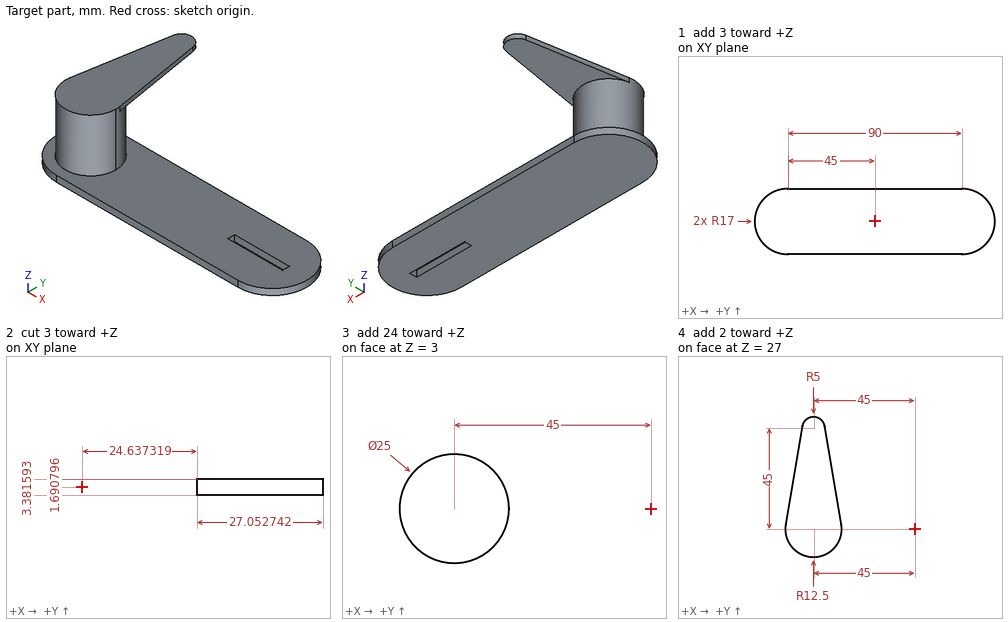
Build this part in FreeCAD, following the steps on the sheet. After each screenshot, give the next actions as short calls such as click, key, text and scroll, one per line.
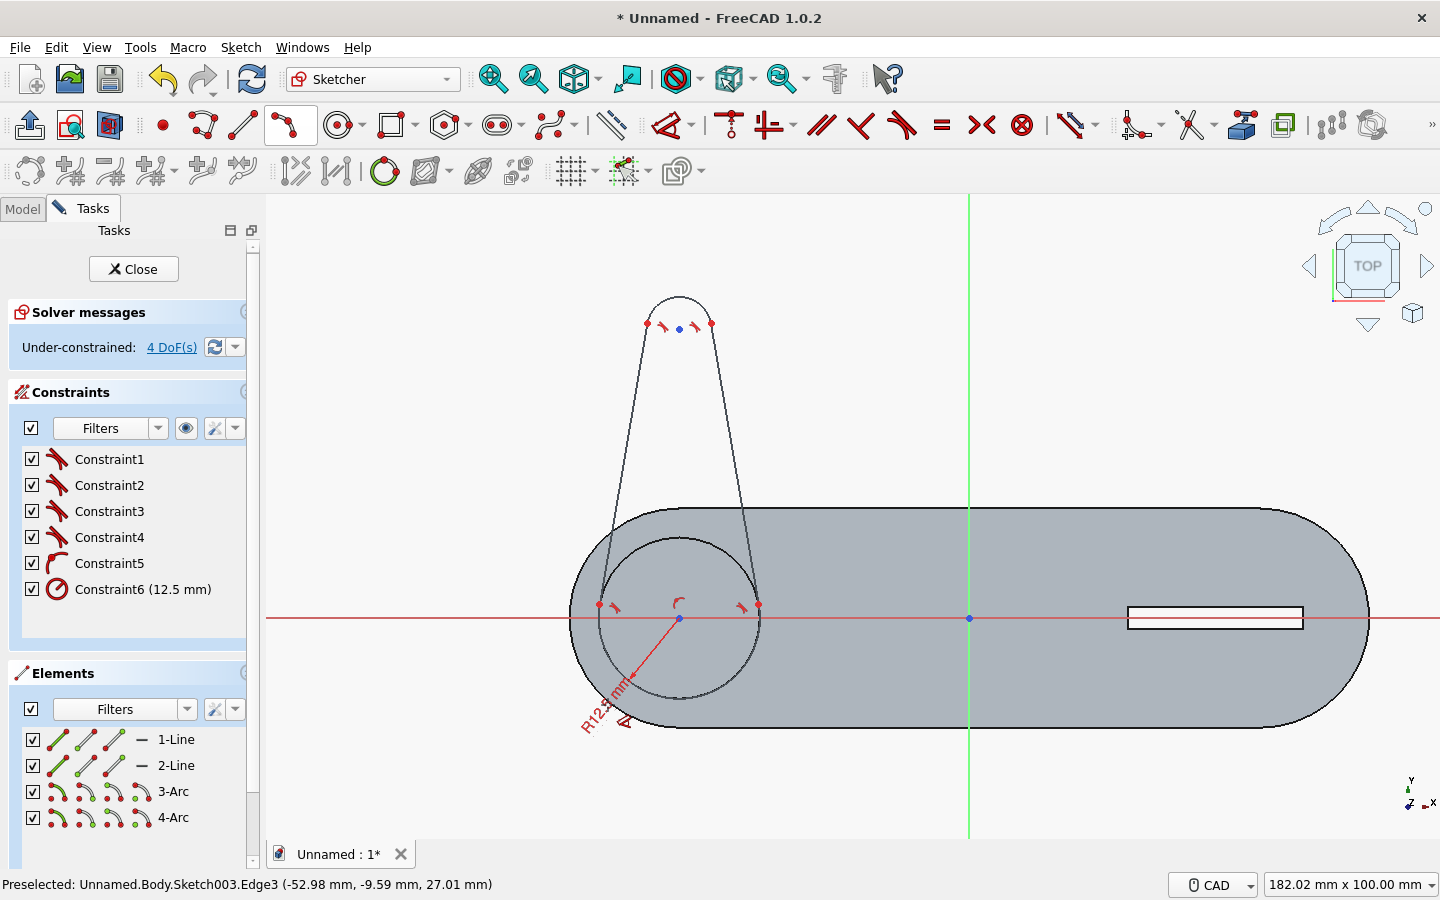
scroll(696, 302, up, 2)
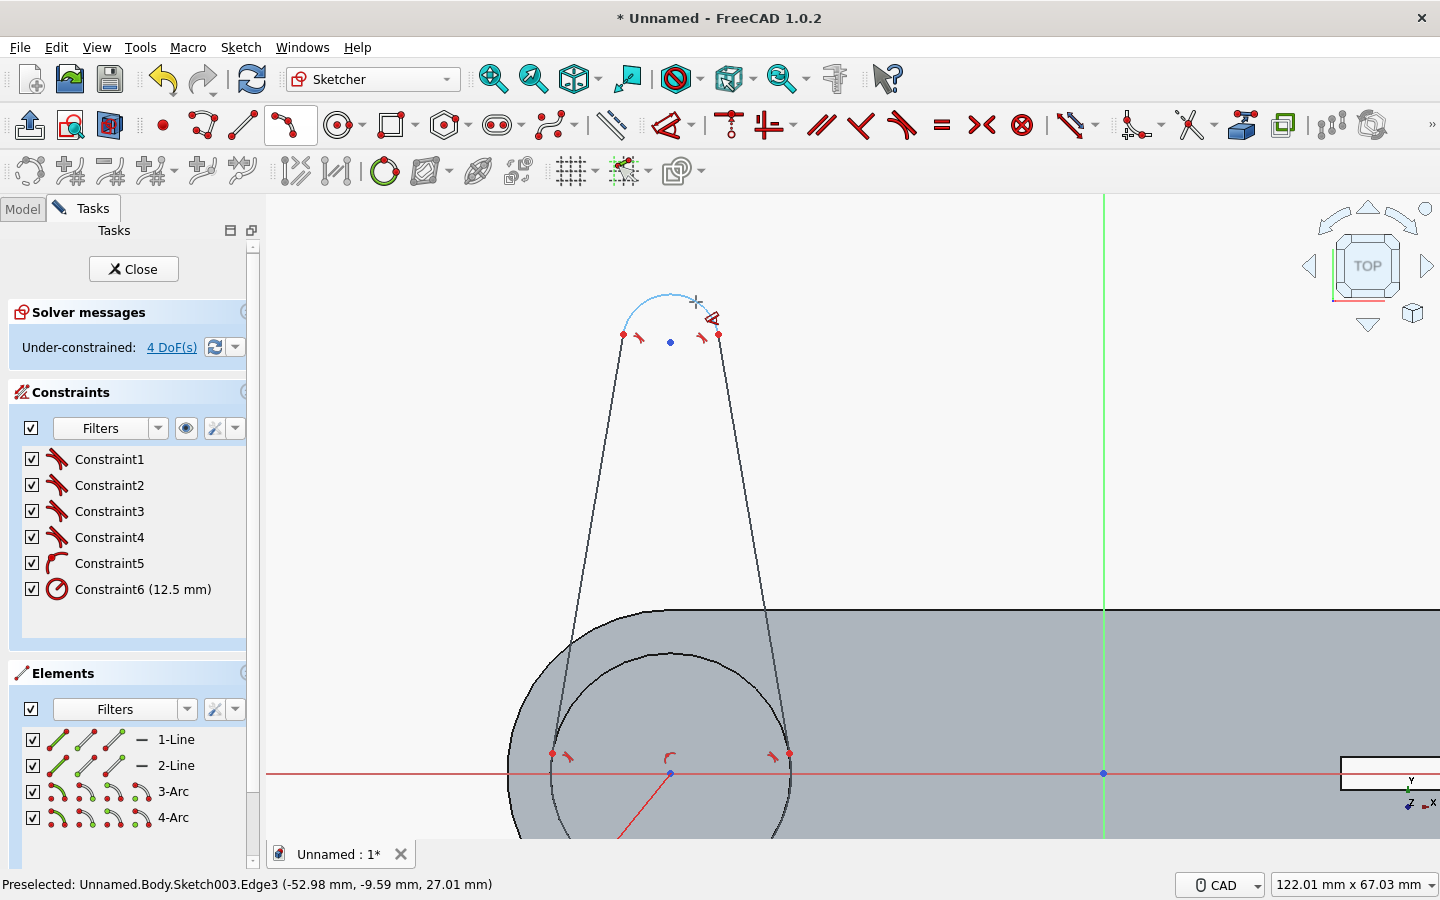
click(696, 302)
click(713, 275)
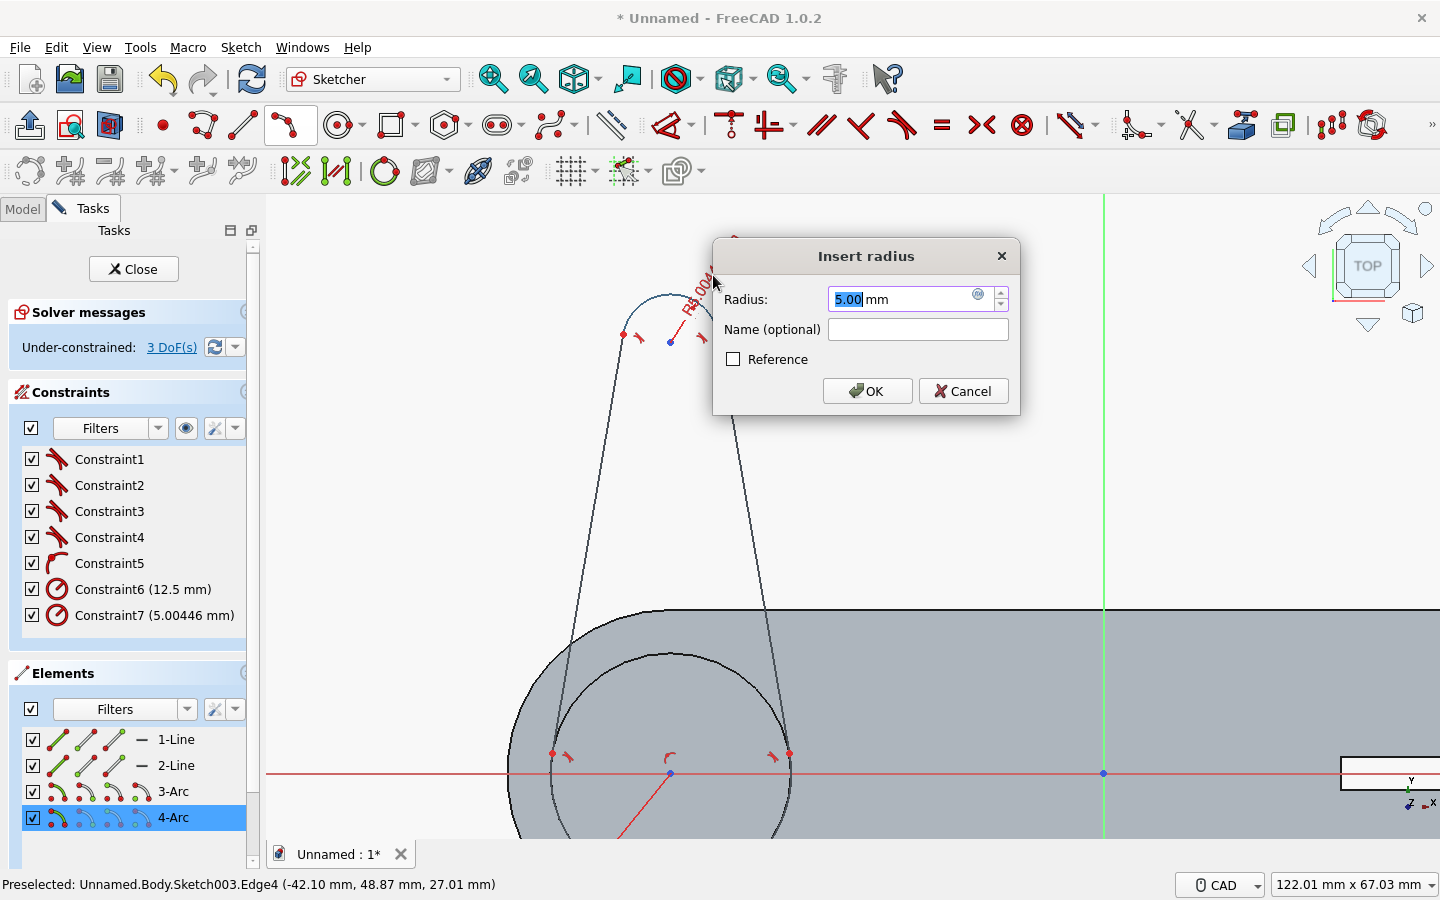
text(5)
key(Return)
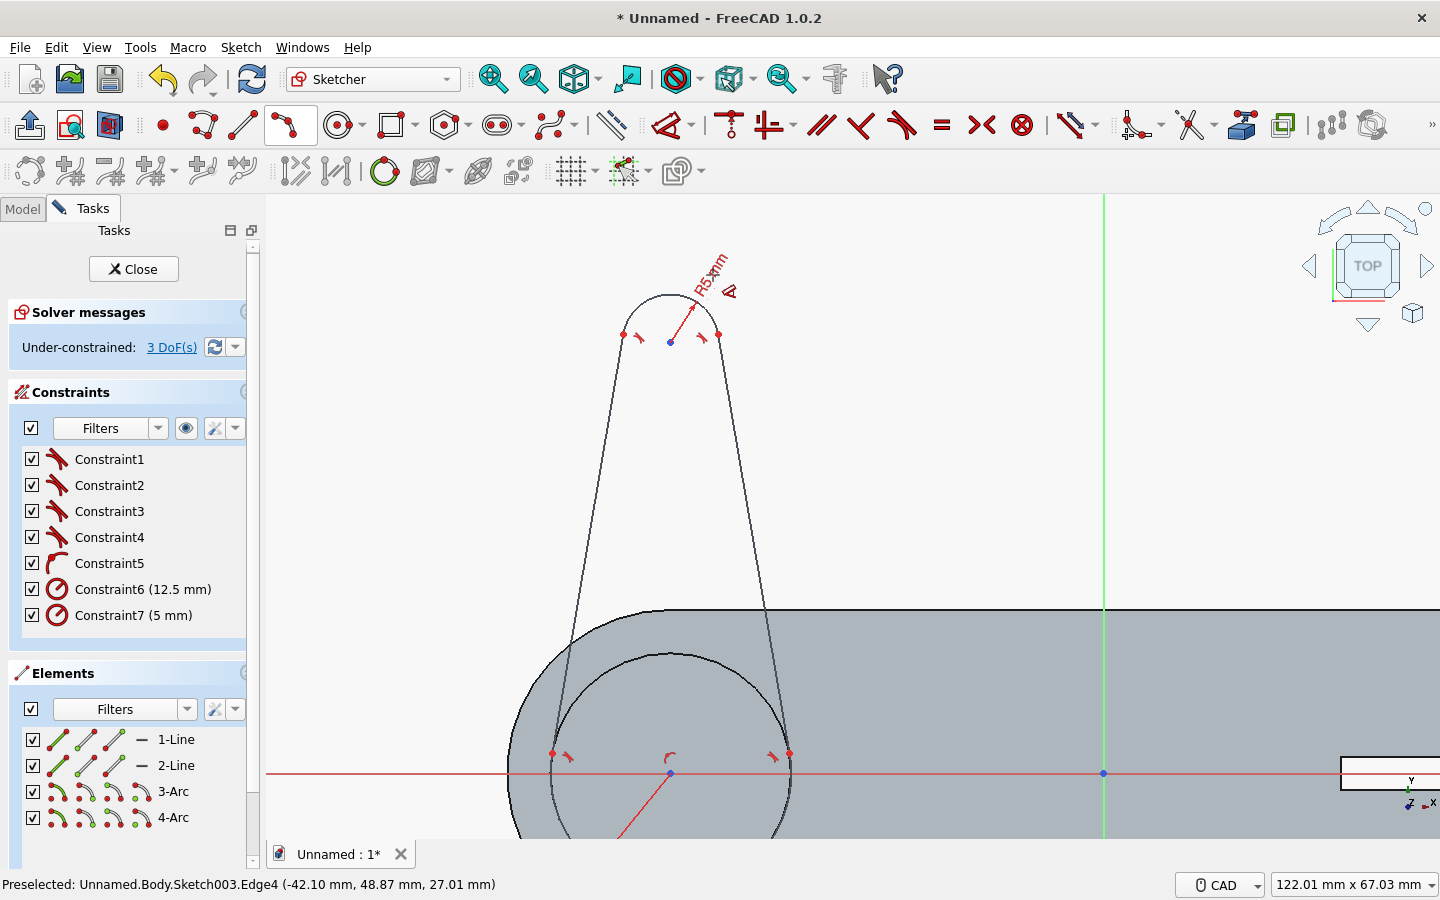
click(671, 774)
click(887, 808)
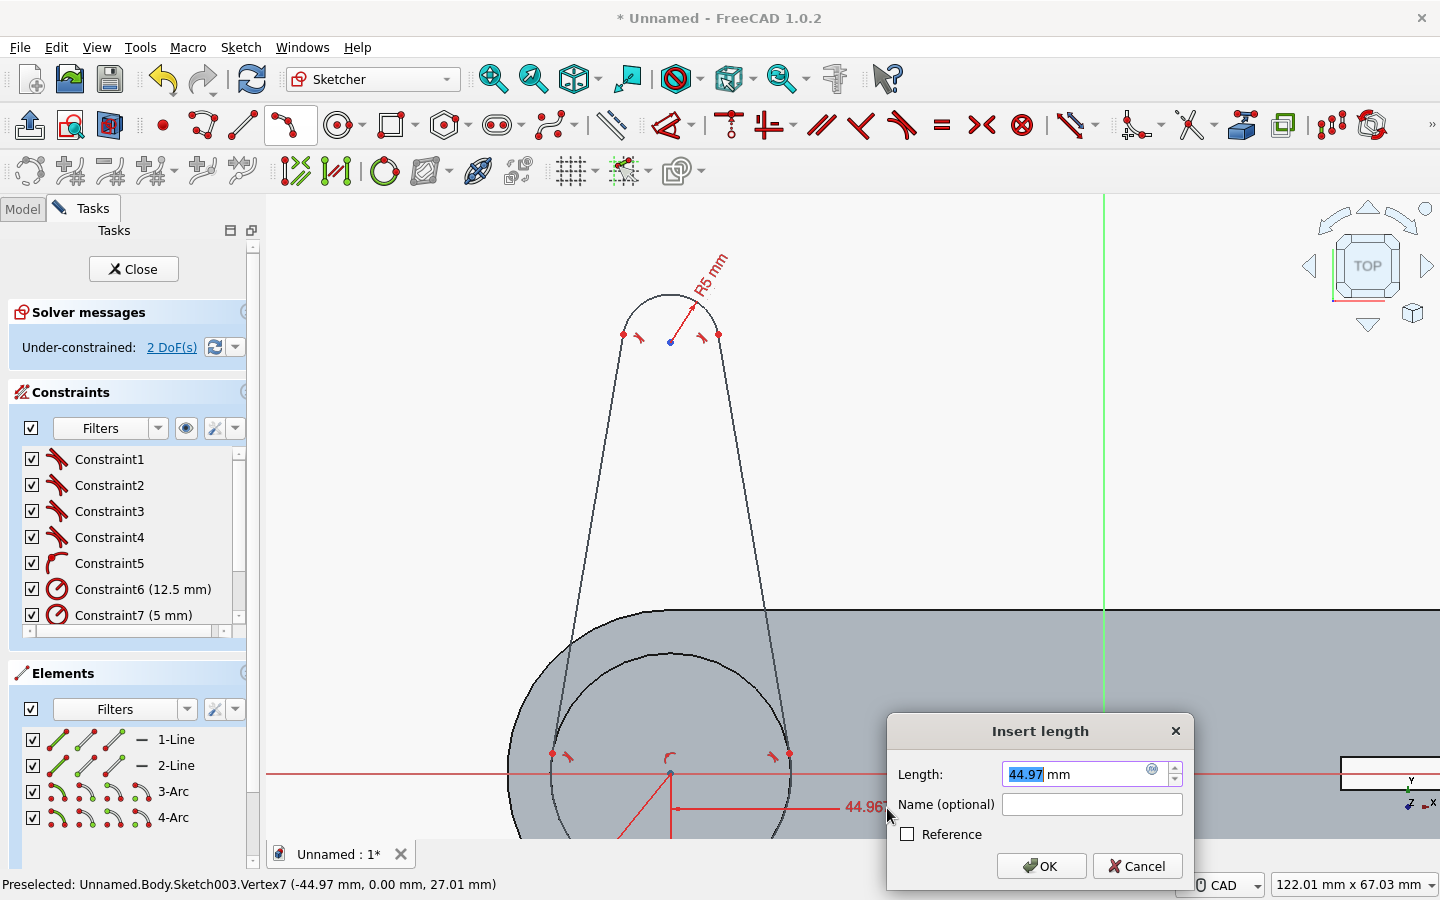
text(45)
key(Return)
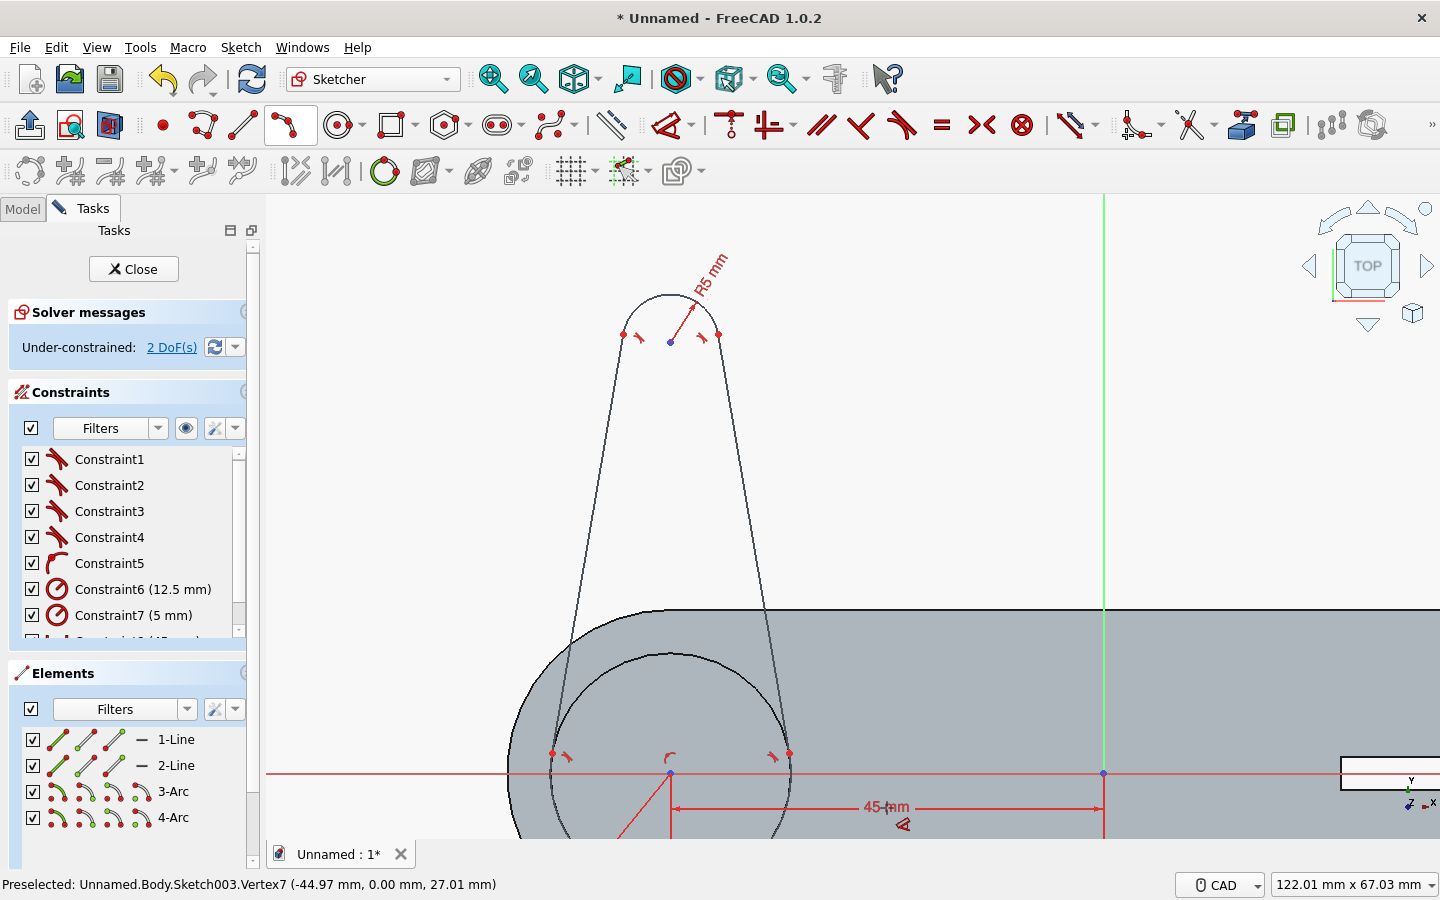
click(671, 343)
click(887, 309)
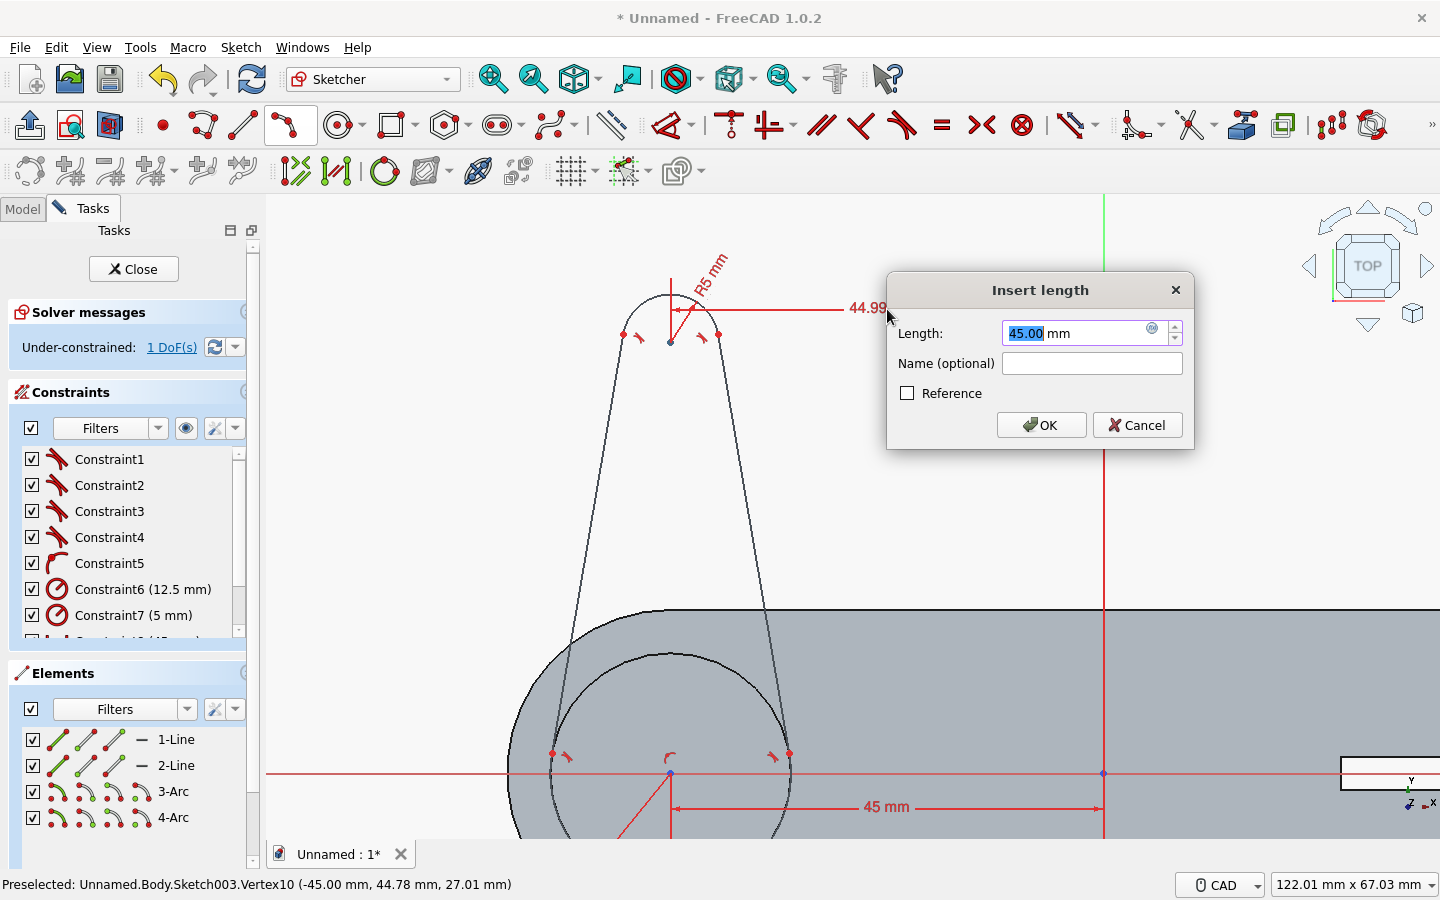
text(45)
key(Return)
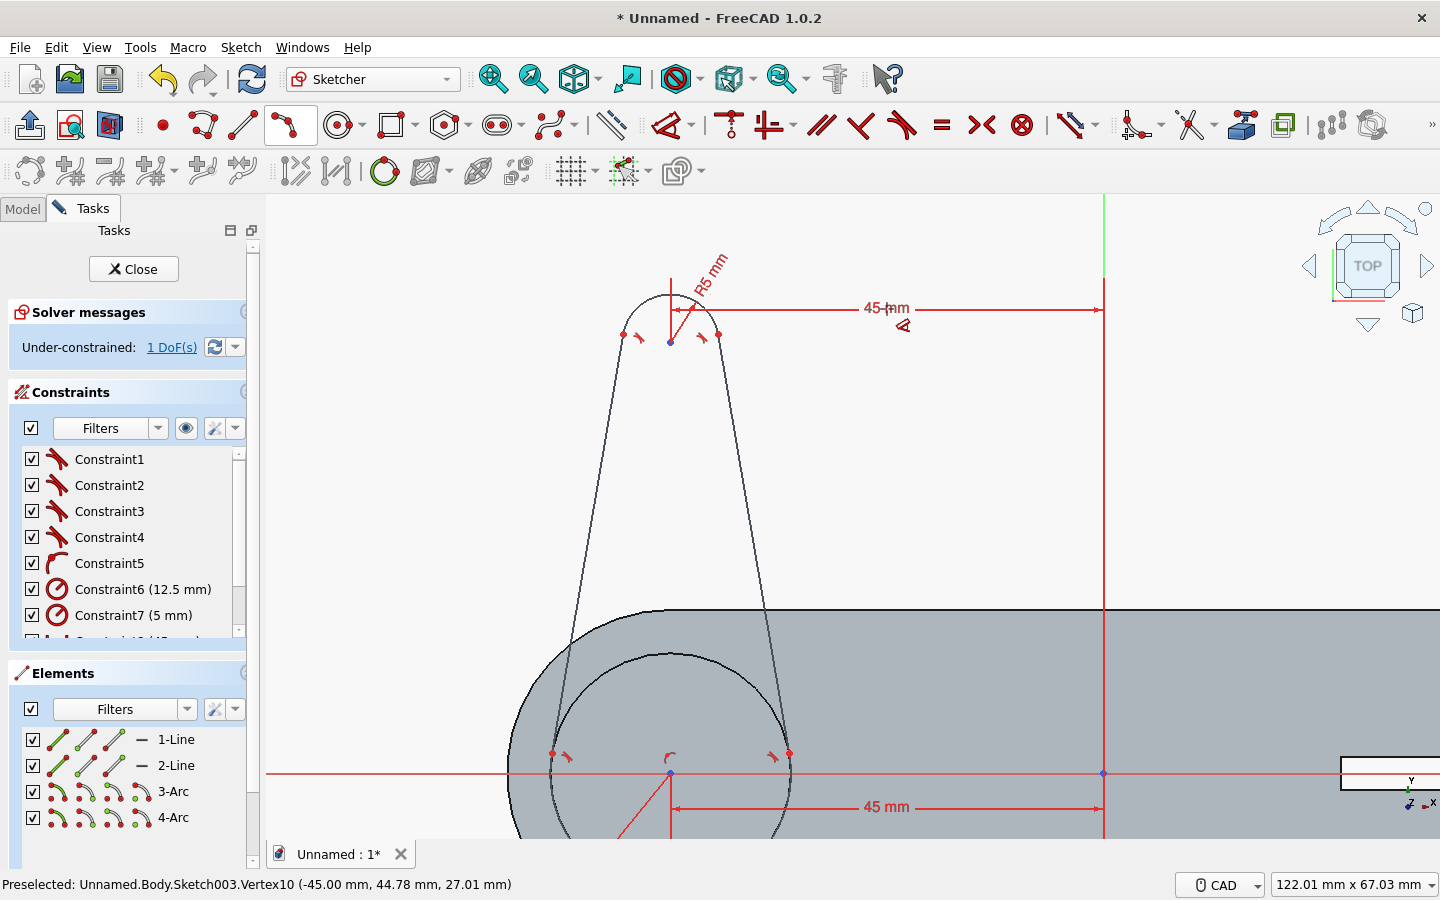
click(671, 343)
click(1138, 558)